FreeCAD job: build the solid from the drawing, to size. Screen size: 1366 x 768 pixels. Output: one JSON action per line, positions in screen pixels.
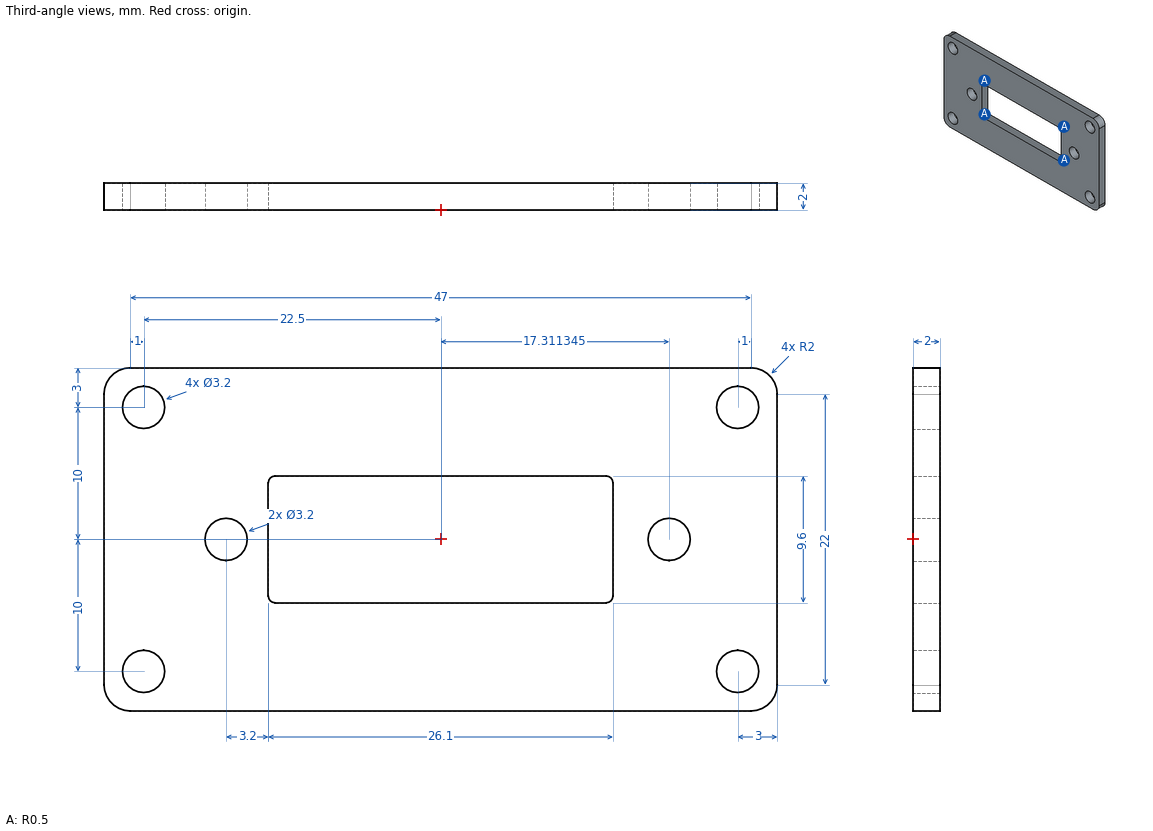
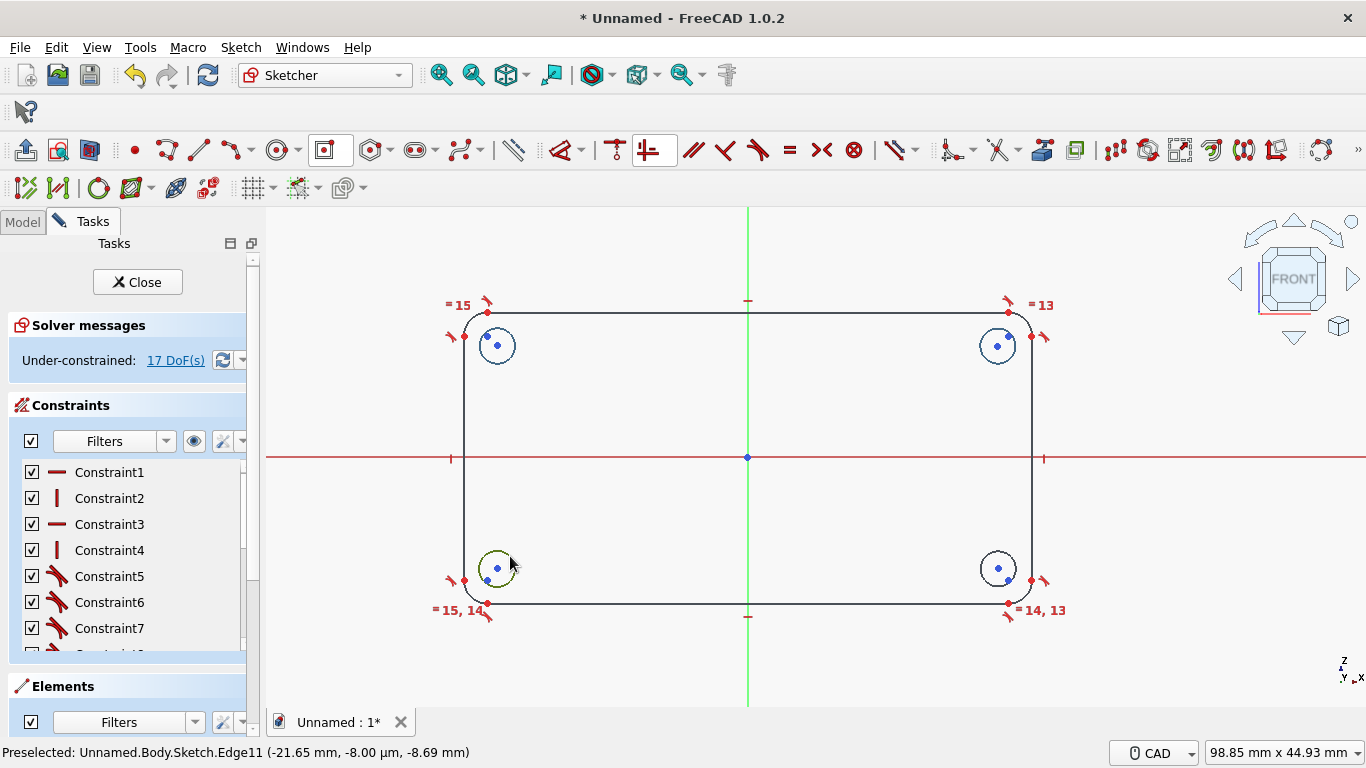
{"action": "left_click", "coordinate": [1011, 556]}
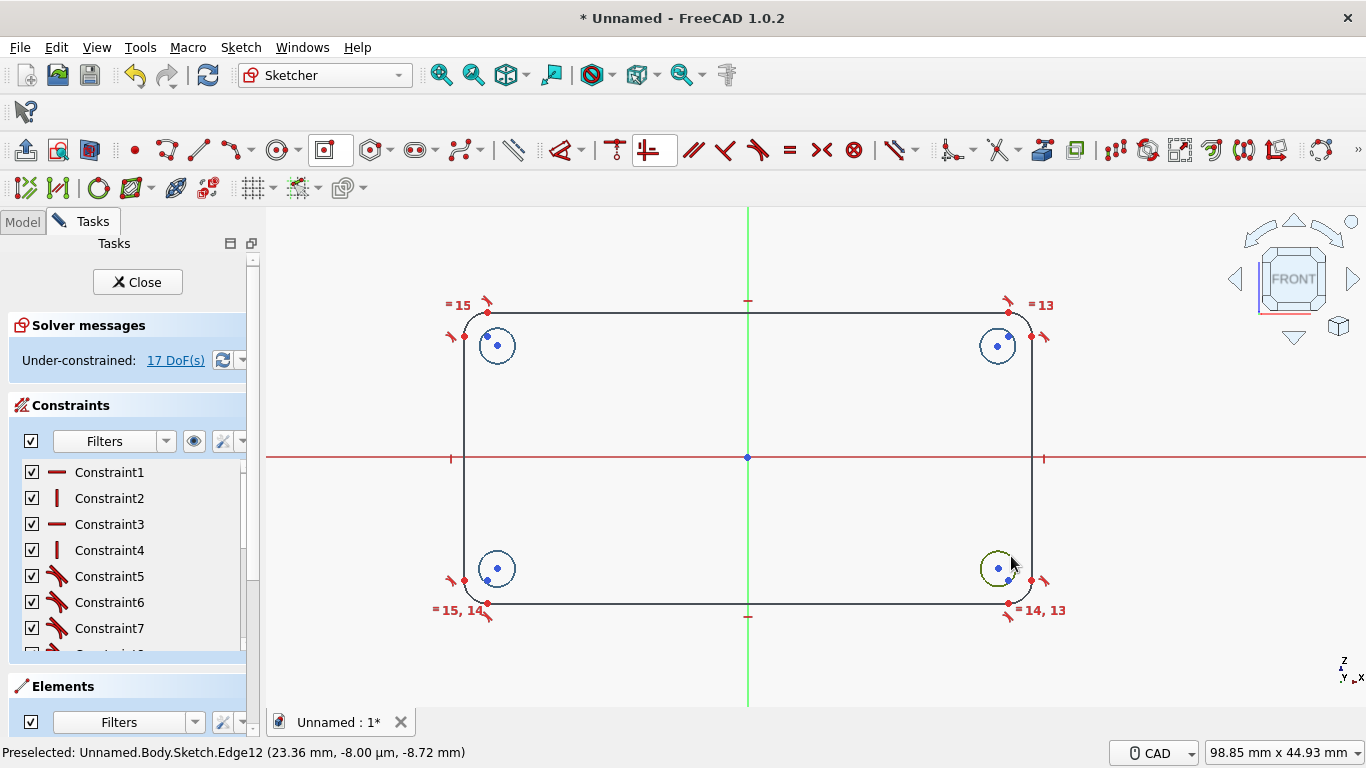
{"action": "left_click", "coordinate": [790, 150]}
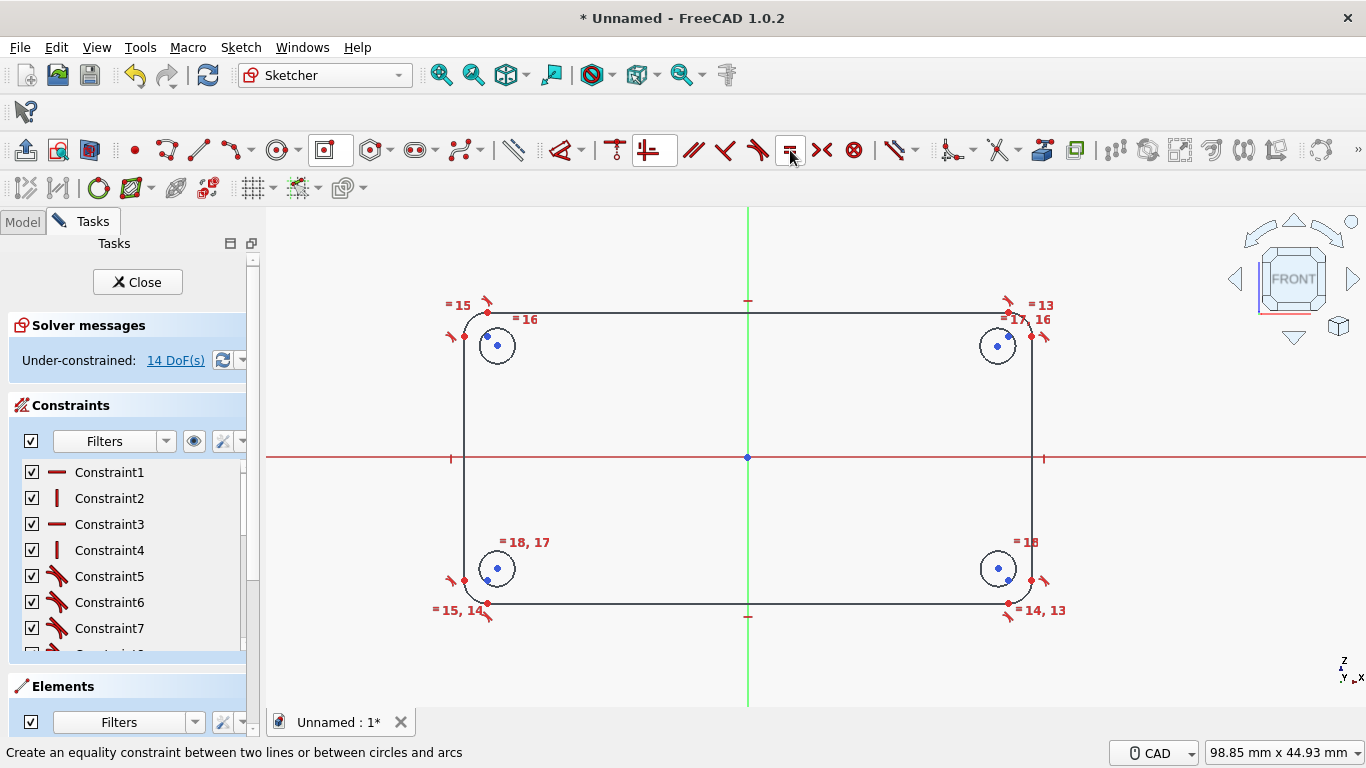
{"action": "left_click", "coordinate": [560, 150]}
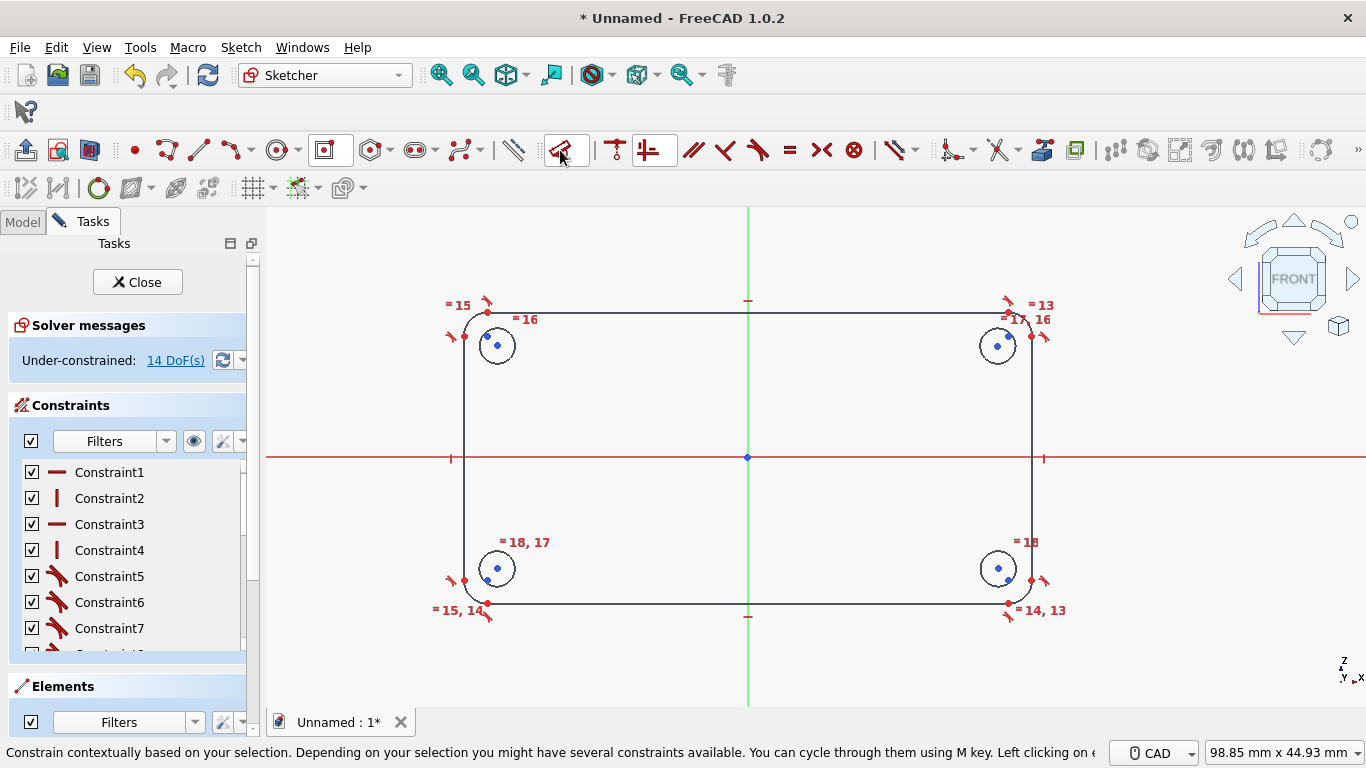
{"action": "scroll", "coordinate": [1029, 325], "scroll_direction": "up", "scroll_amount": 3}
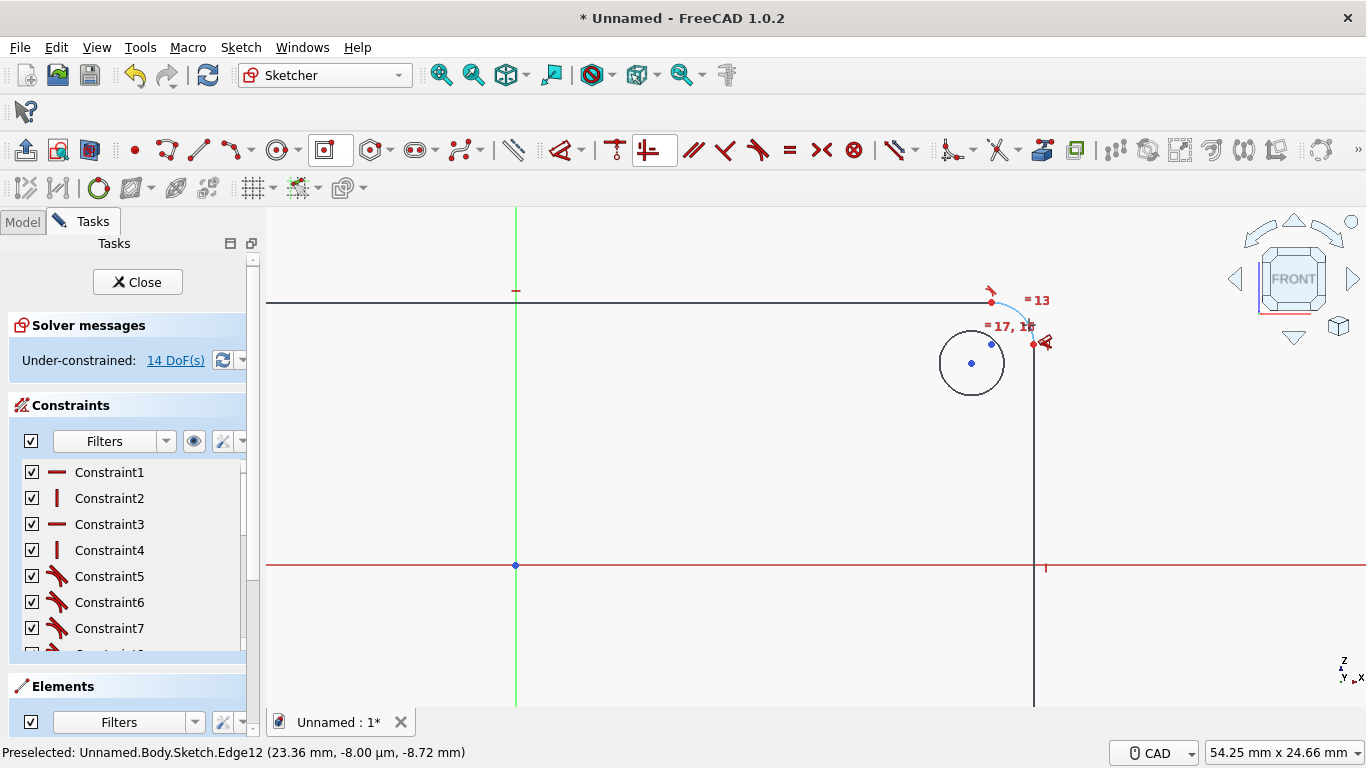
{"action": "left_click", "coordinate": [1029, 326]}
{"action": "left_click", "coordinate": [1058, 312]}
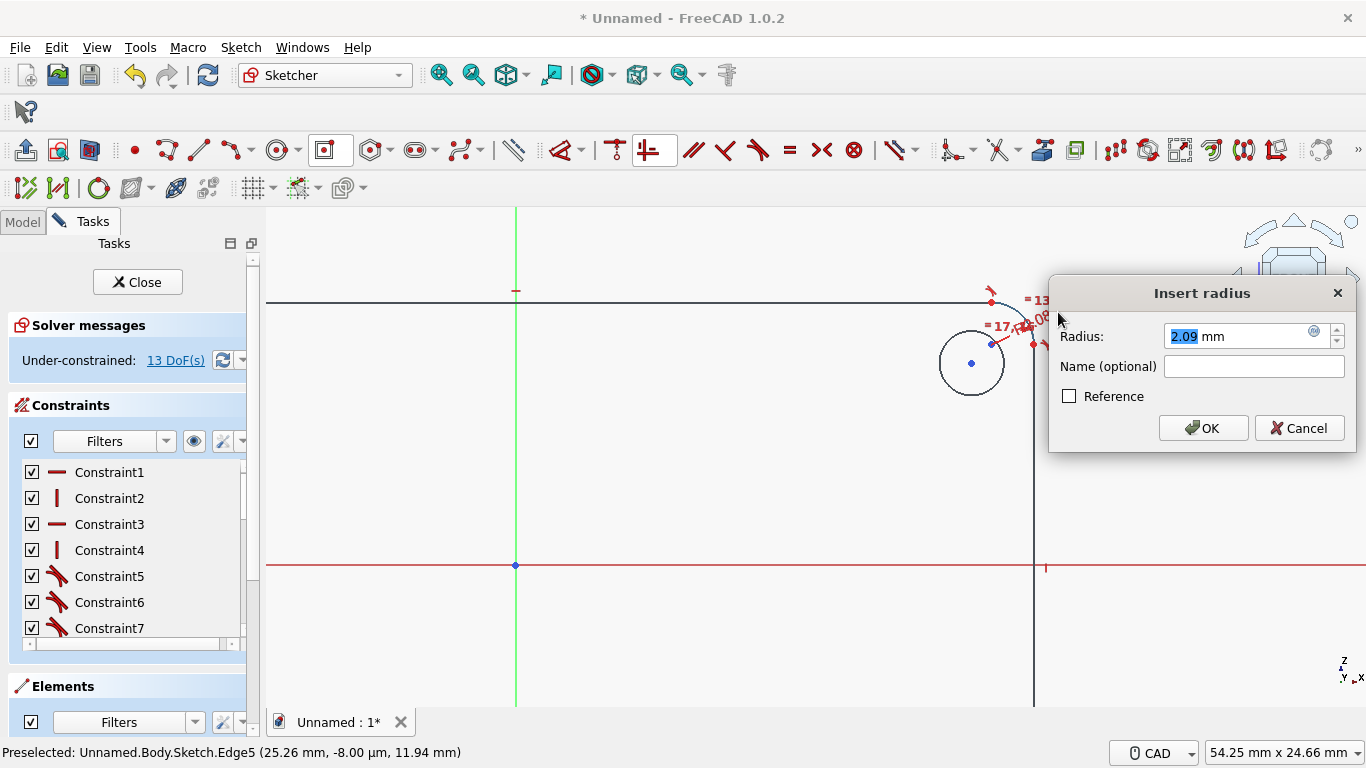
{"action": "type", "text": "2"}
{"action": "key", "text": "Return"}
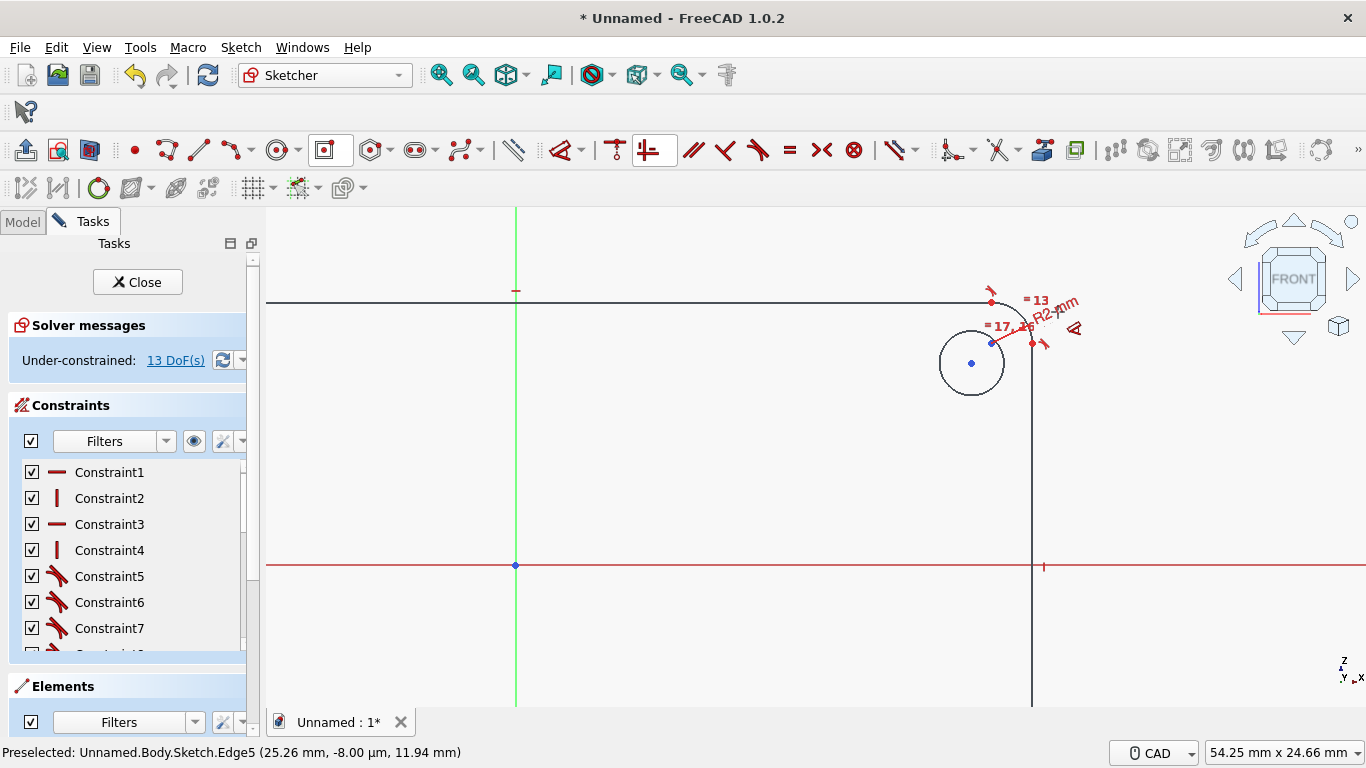
{"action": "scroll", "coordinate": [1029, 325], "scroll_direction": "down", "scroll_amount": 3}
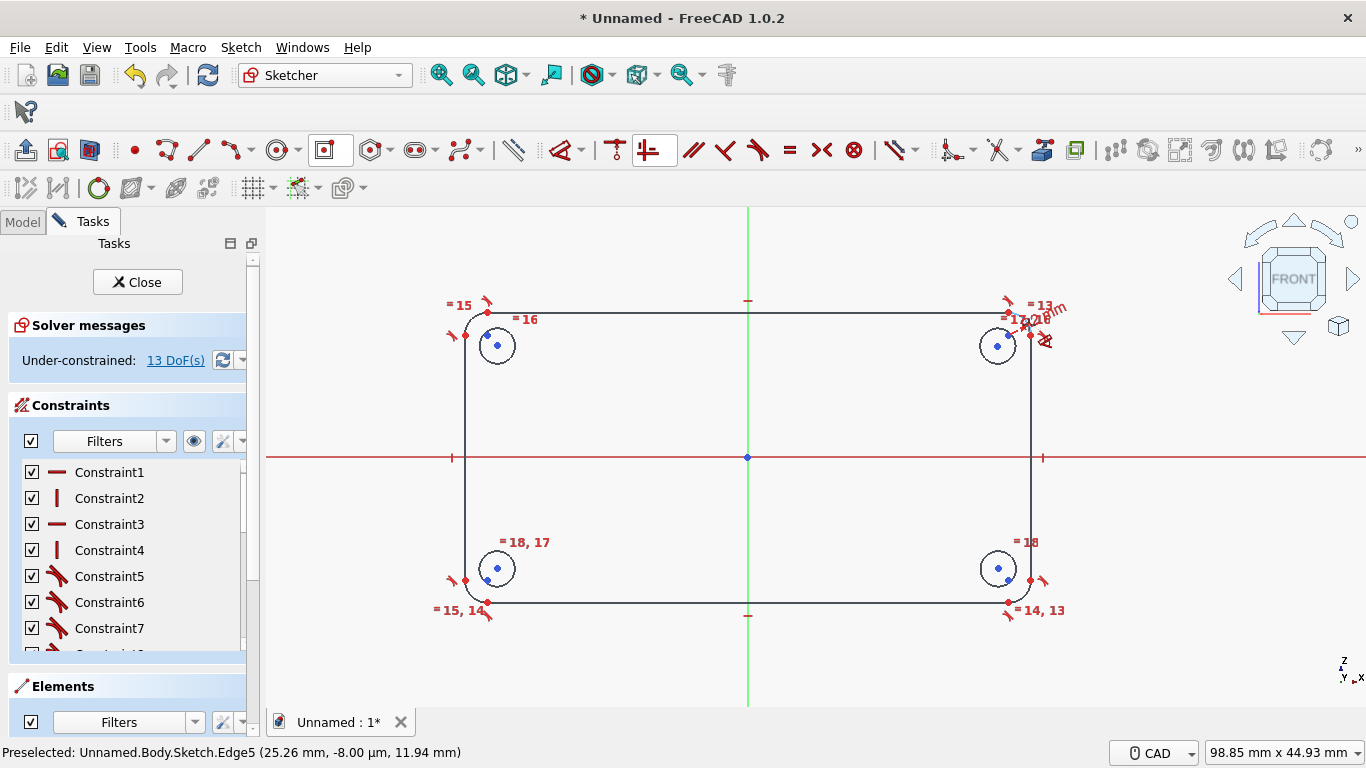
{"action": "left_click", "coordinate": [510, 333]}
{"action": "left_click", "coordinate": [545, 331]}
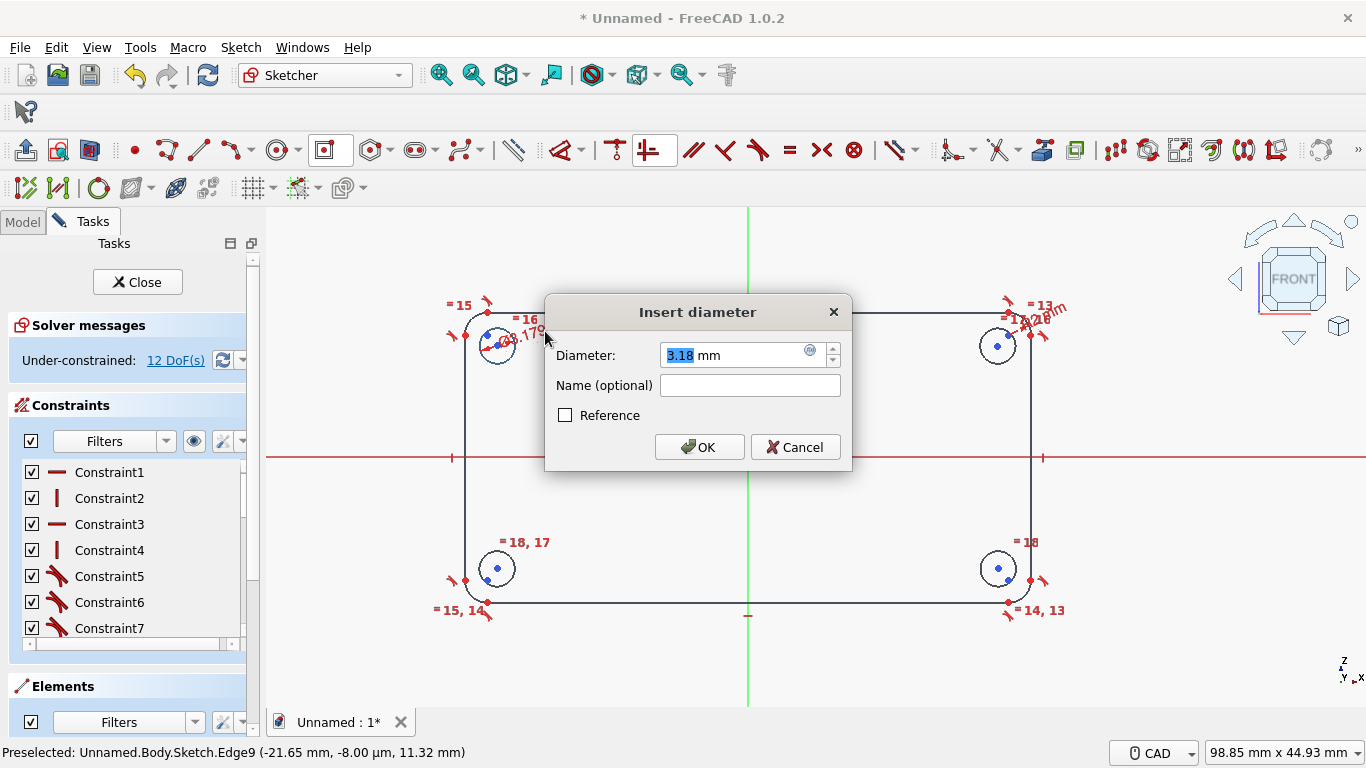
{"action": "type", "text": "3.2"}
{"action": "key", "text": "Return"}